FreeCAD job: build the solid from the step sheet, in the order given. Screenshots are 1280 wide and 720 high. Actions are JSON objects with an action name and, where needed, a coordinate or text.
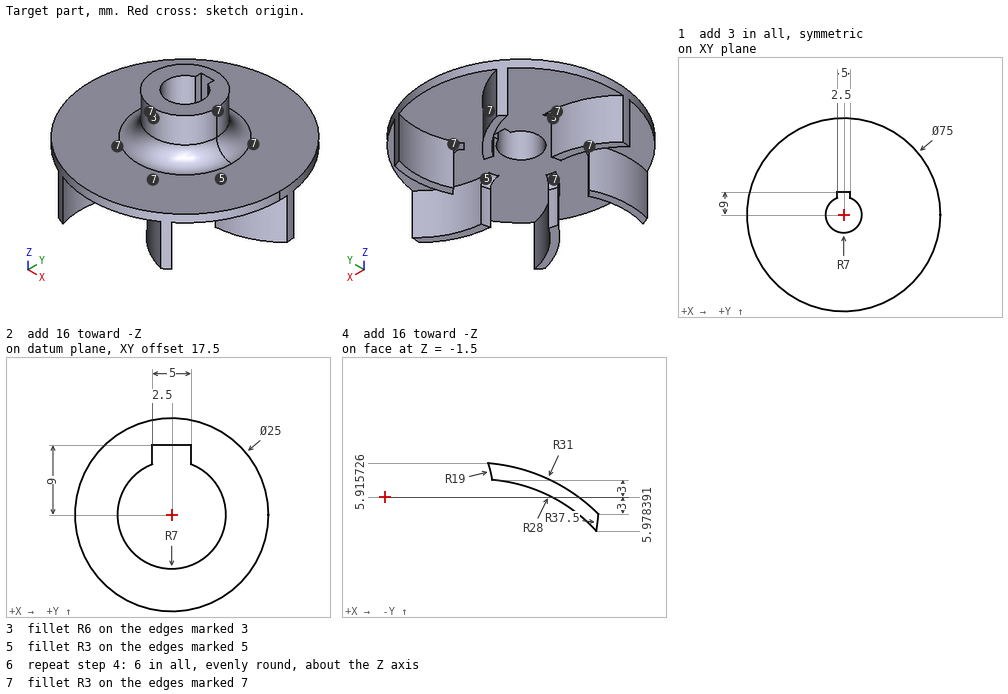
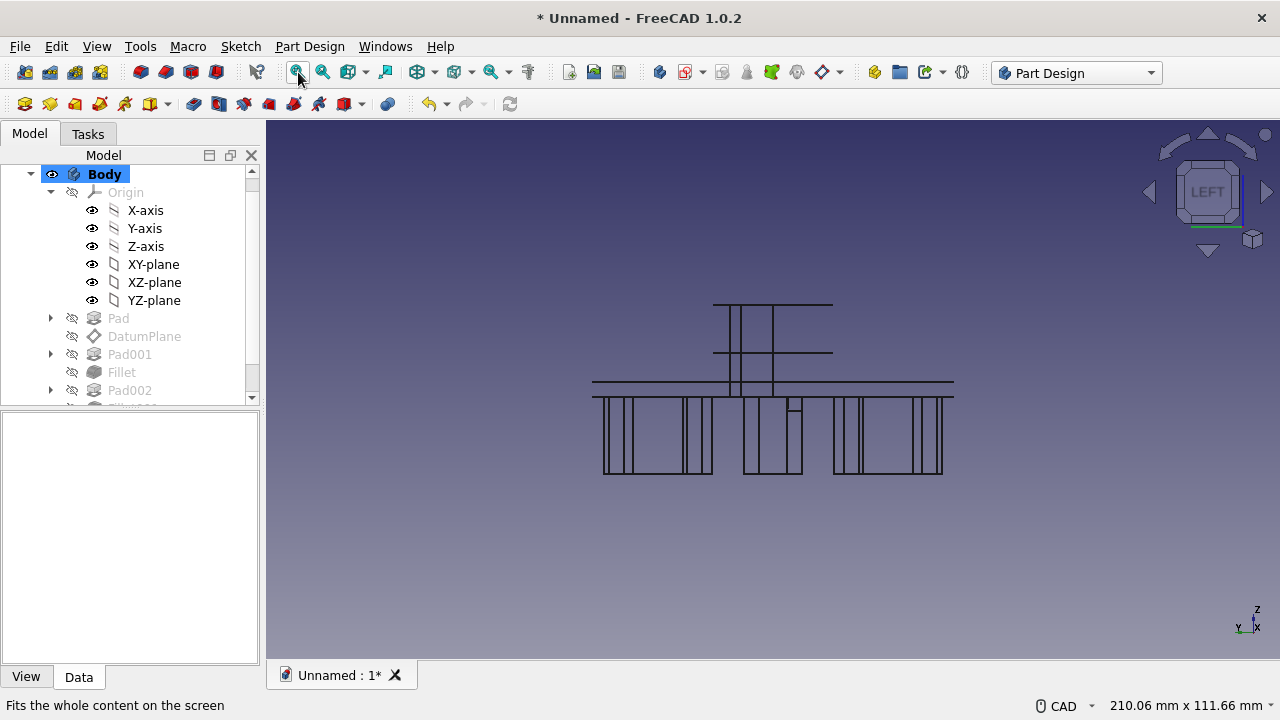
{"action": "key", "text": "0"}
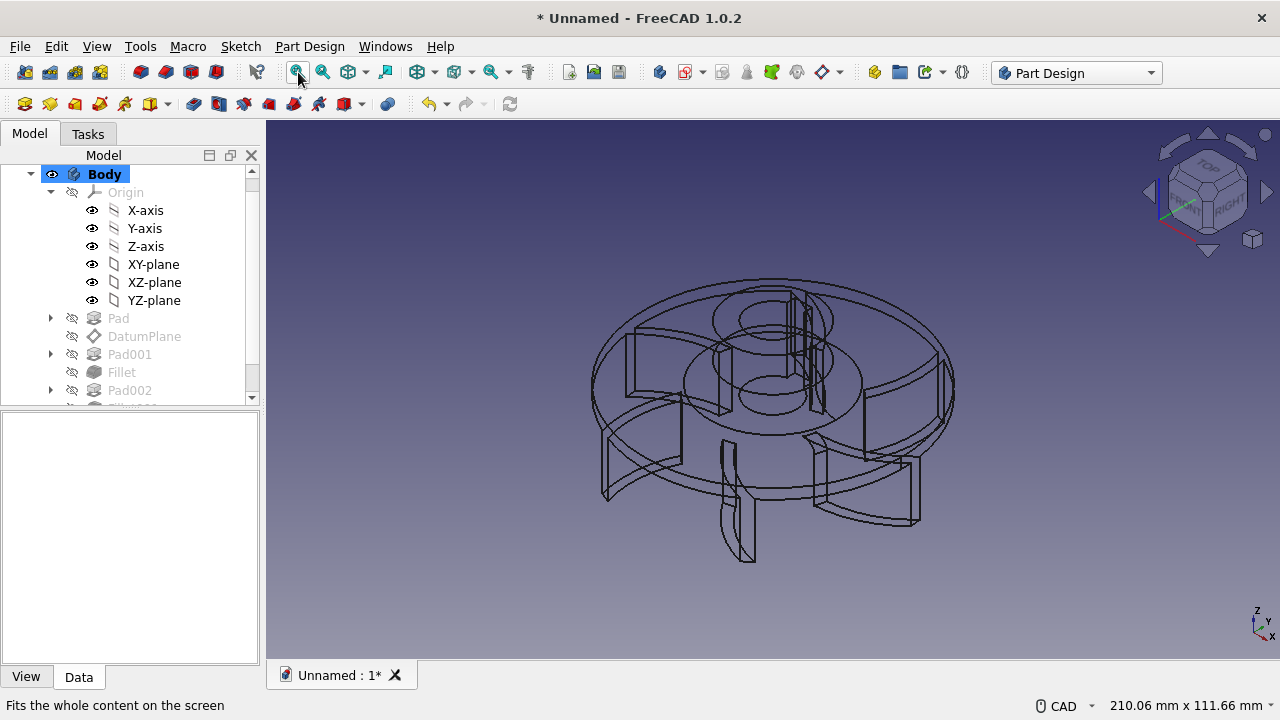
{"action": "left_click", "coordinate": [725, 349]}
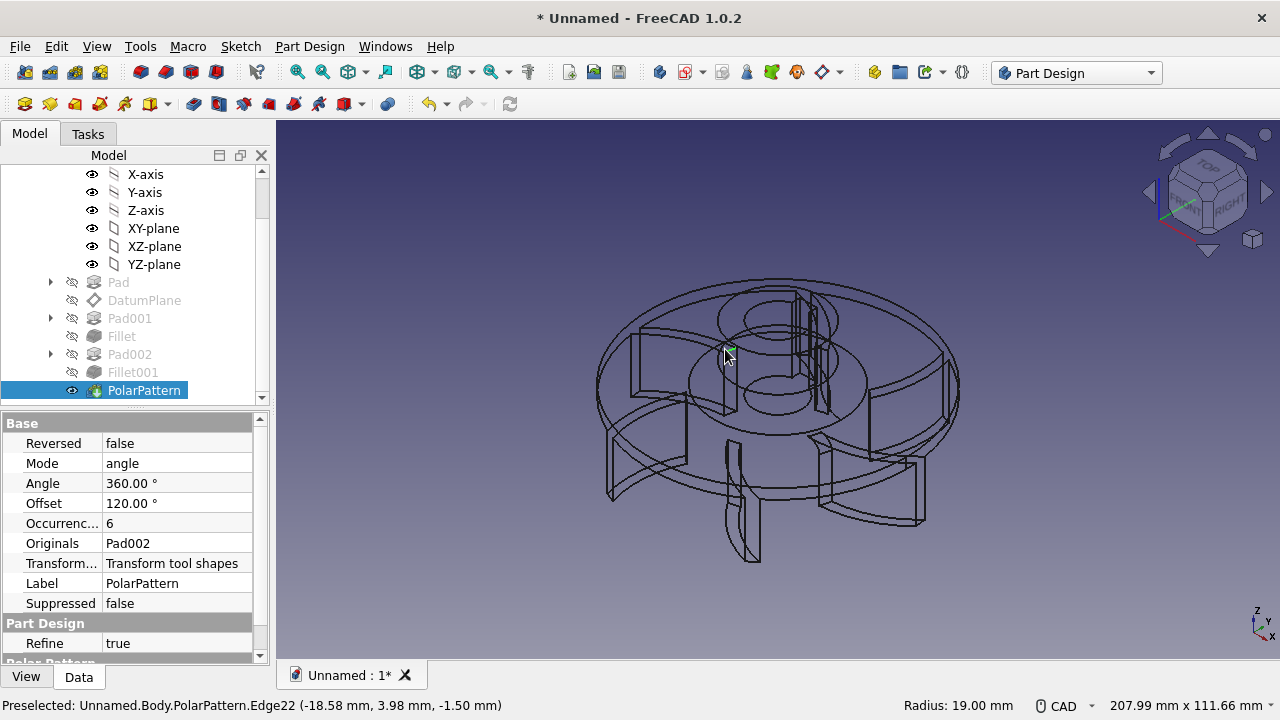
{"action": "left_click", "coordinate": [734, 441], "text": "ctrl"}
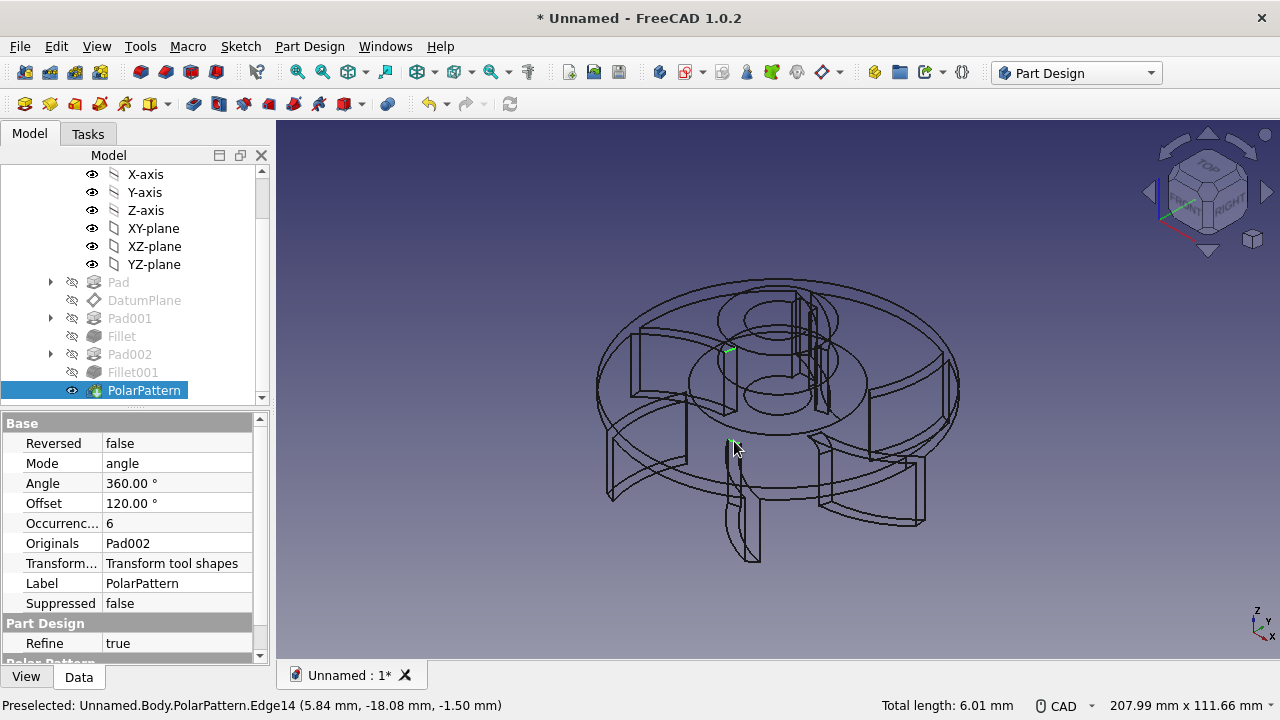
{"action": "scroll", "coordinate": [870, 393], "scroll_direction": "up", "scroll_amount": 6}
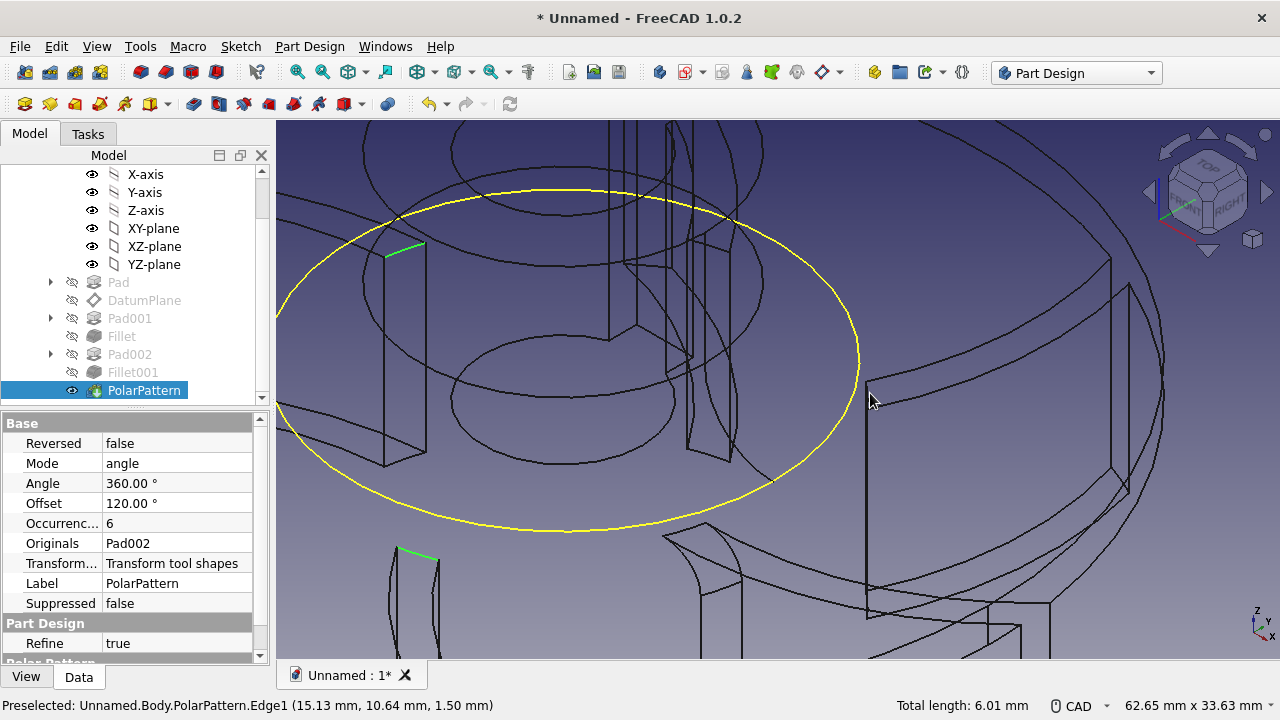
{"action": "left_click", "coordinate": [868, 395], "text": "ctrl"}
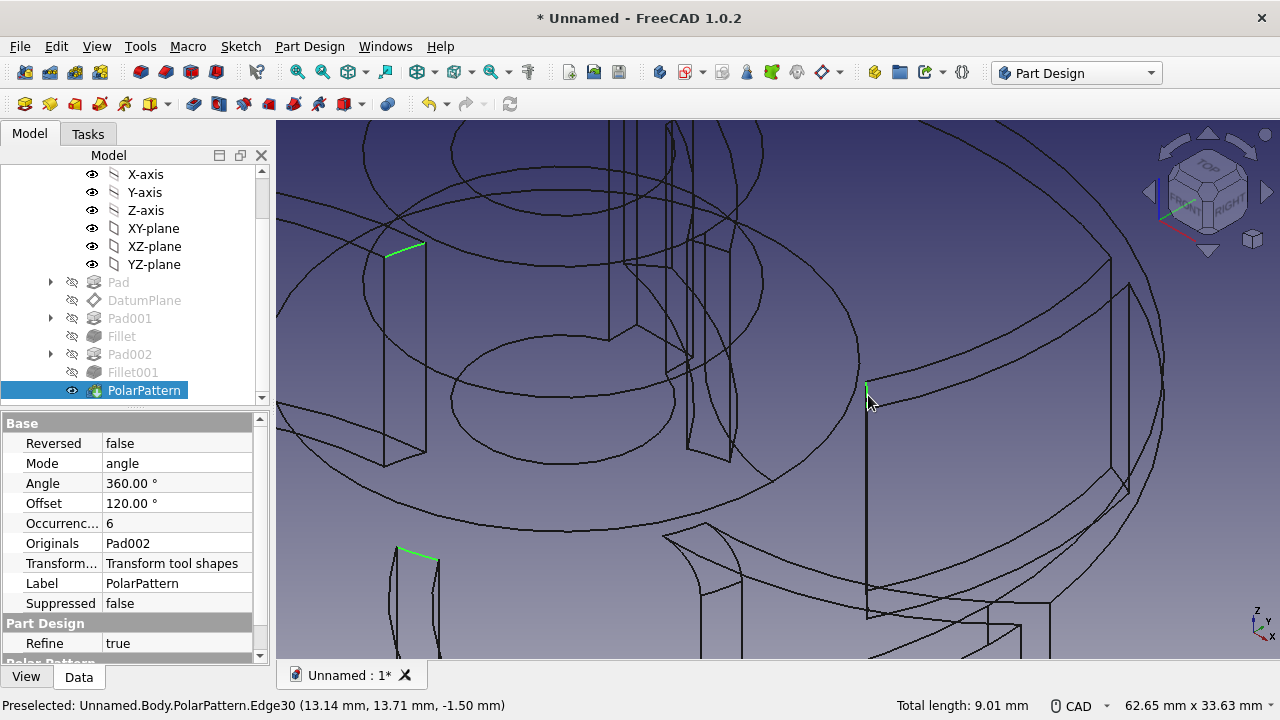
{"action": "left_click", "coordinate": [713, 246], "text": "ctrl"}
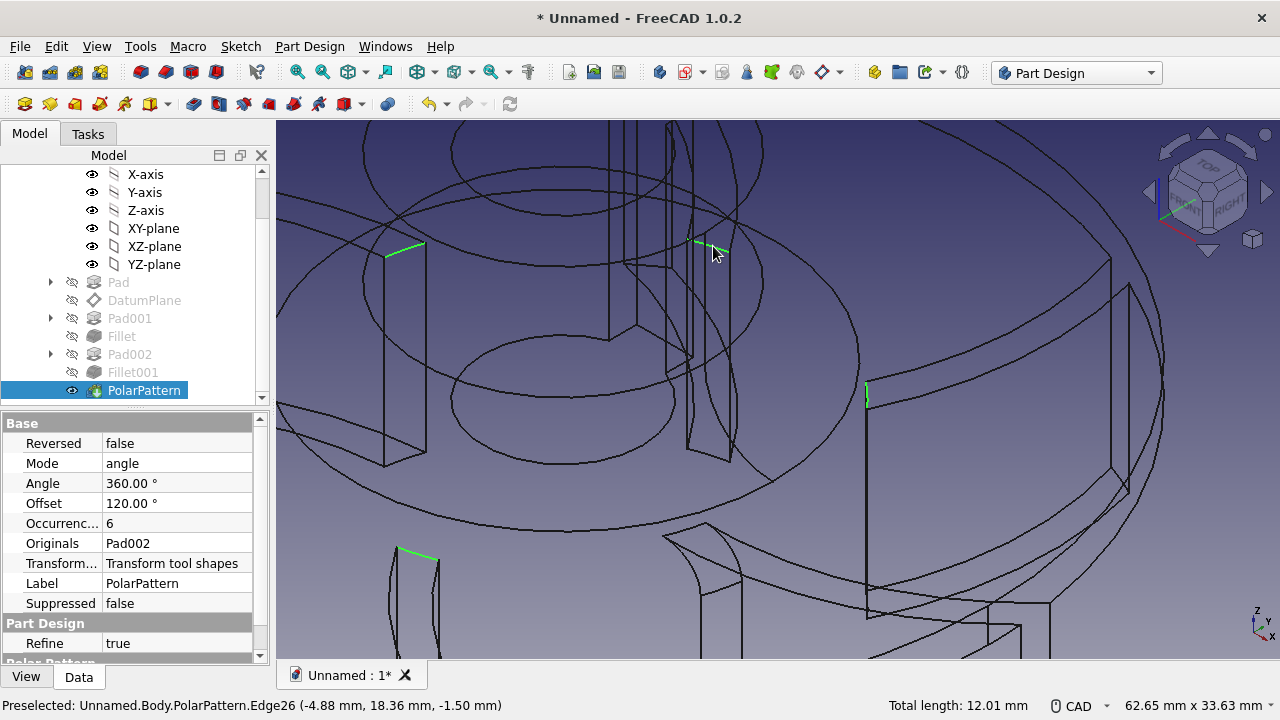
{"action": "left_click", "coordinate": [298, 72]}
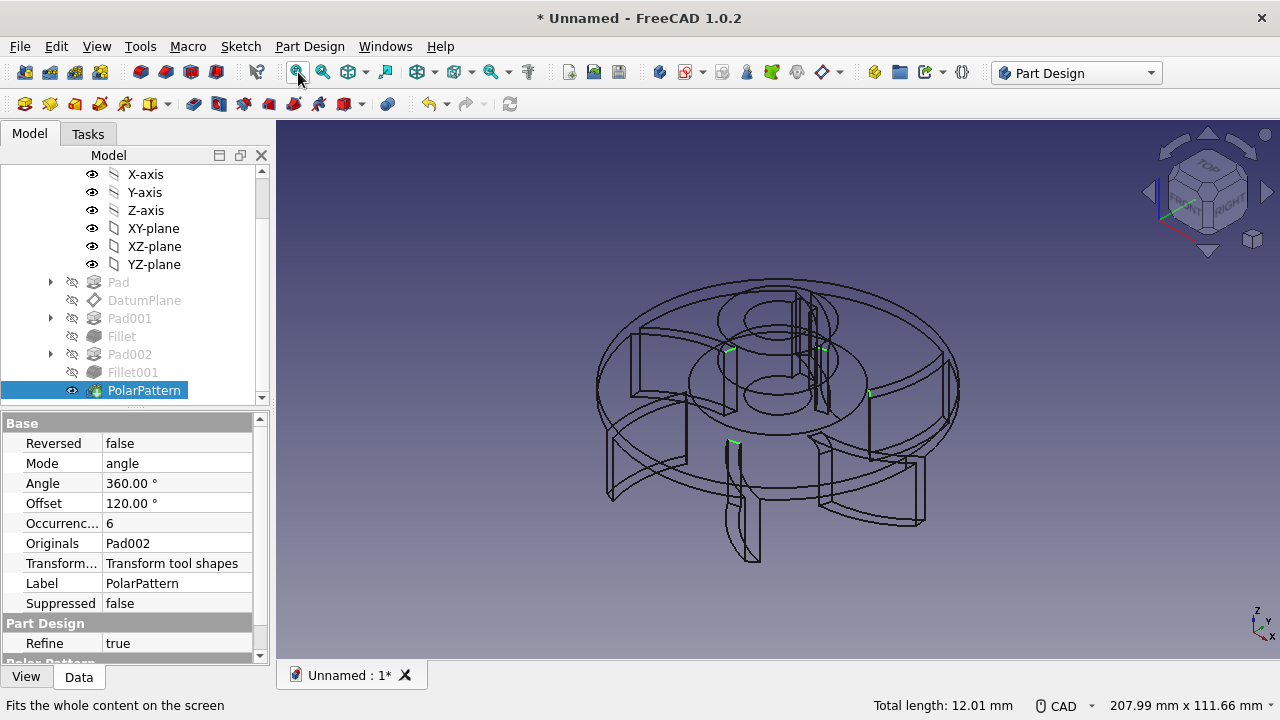
{"action": "key", "text": "2"}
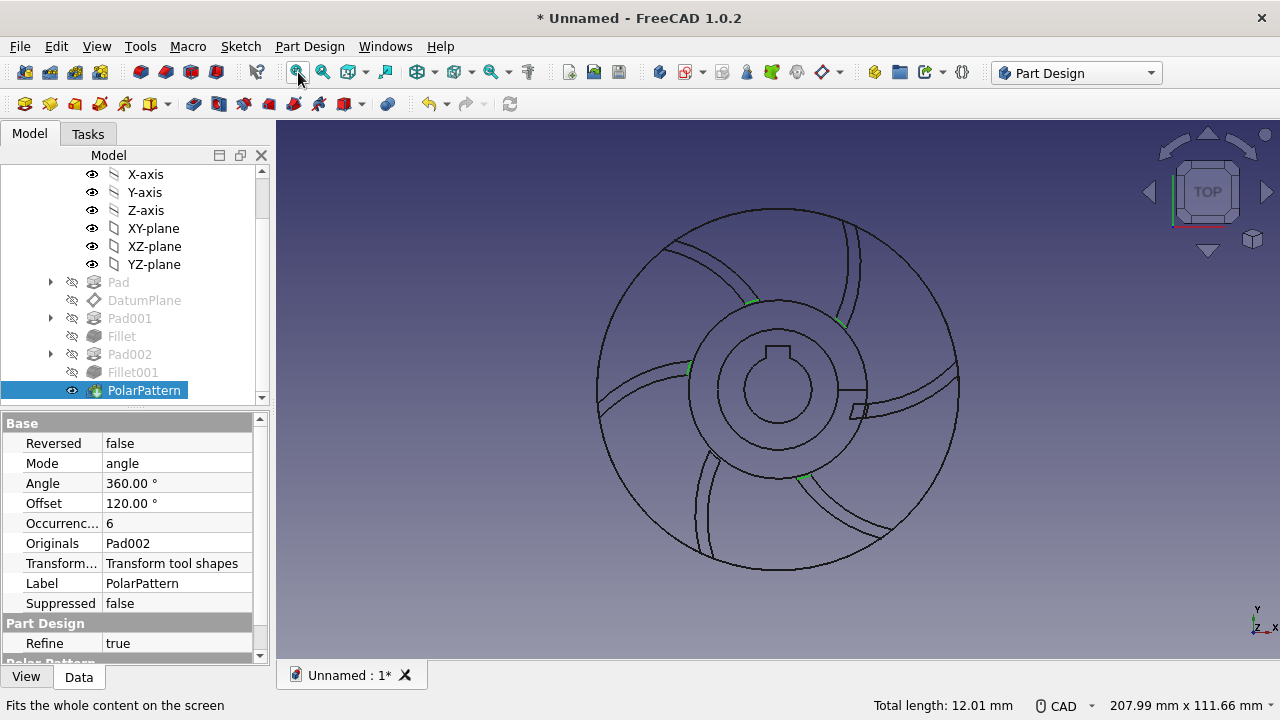
{"action": "scroll", "coordinate": [715, 455], "scroll_direction": "up", "scroll_amount": 6}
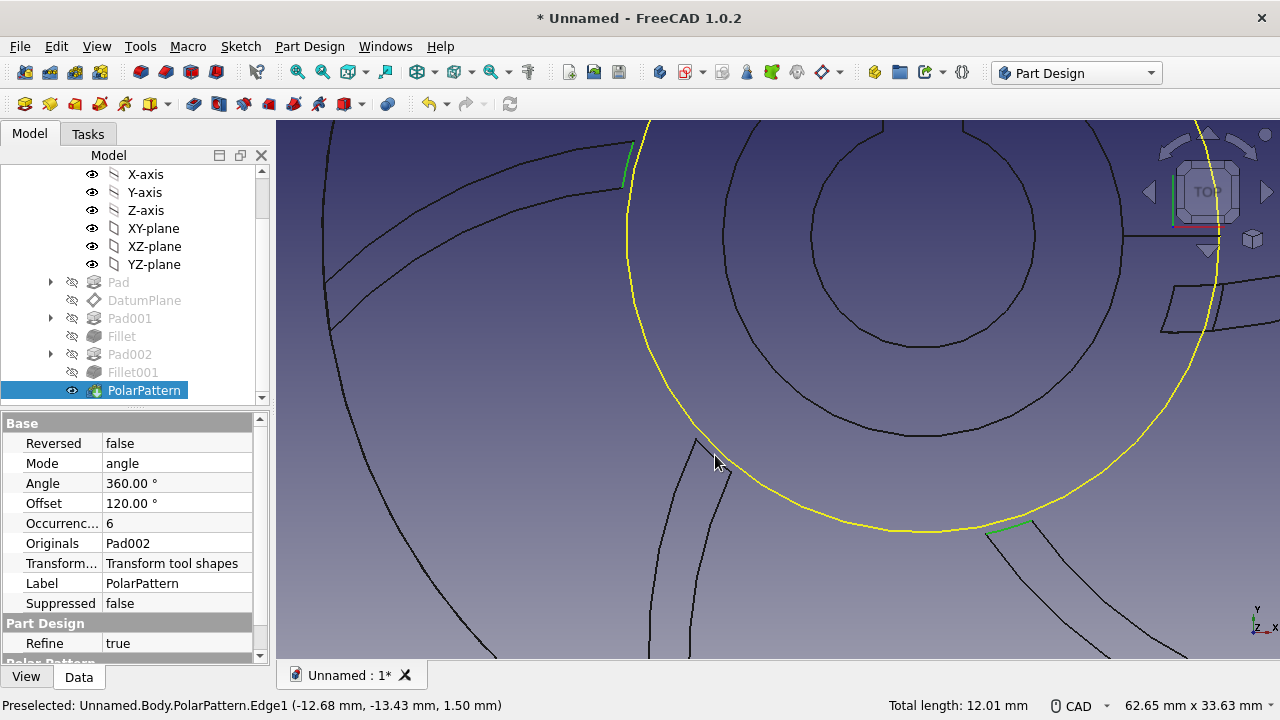
{"action": "left_click", "coordinate": [713, 456], "text": "ctrl"}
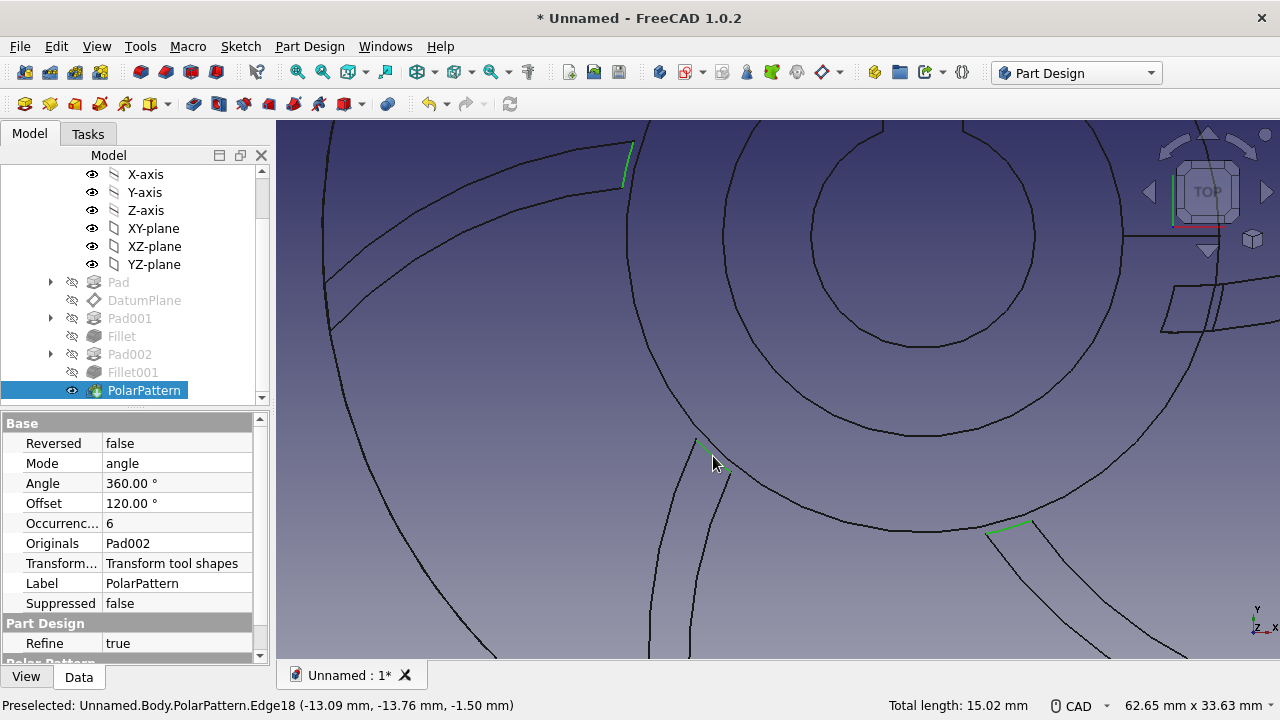
{"action": "key", "text": "v 1"}